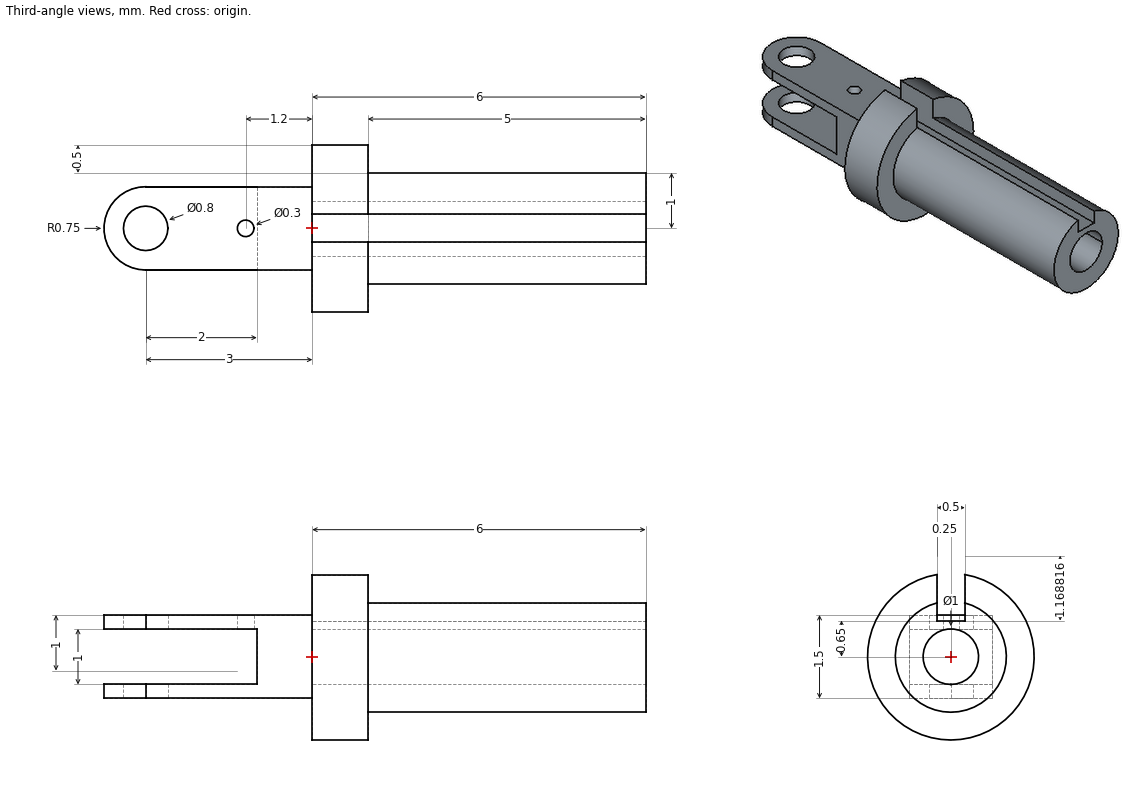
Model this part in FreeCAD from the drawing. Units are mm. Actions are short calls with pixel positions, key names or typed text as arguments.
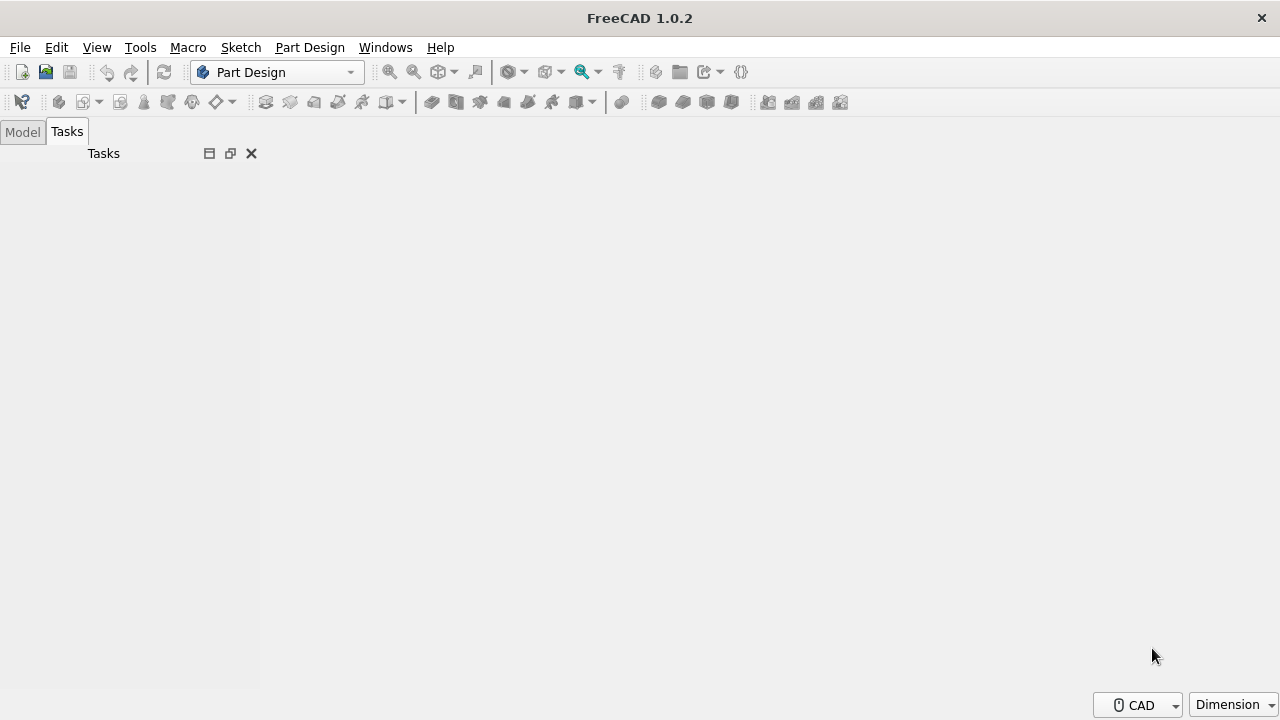
click(22, 72)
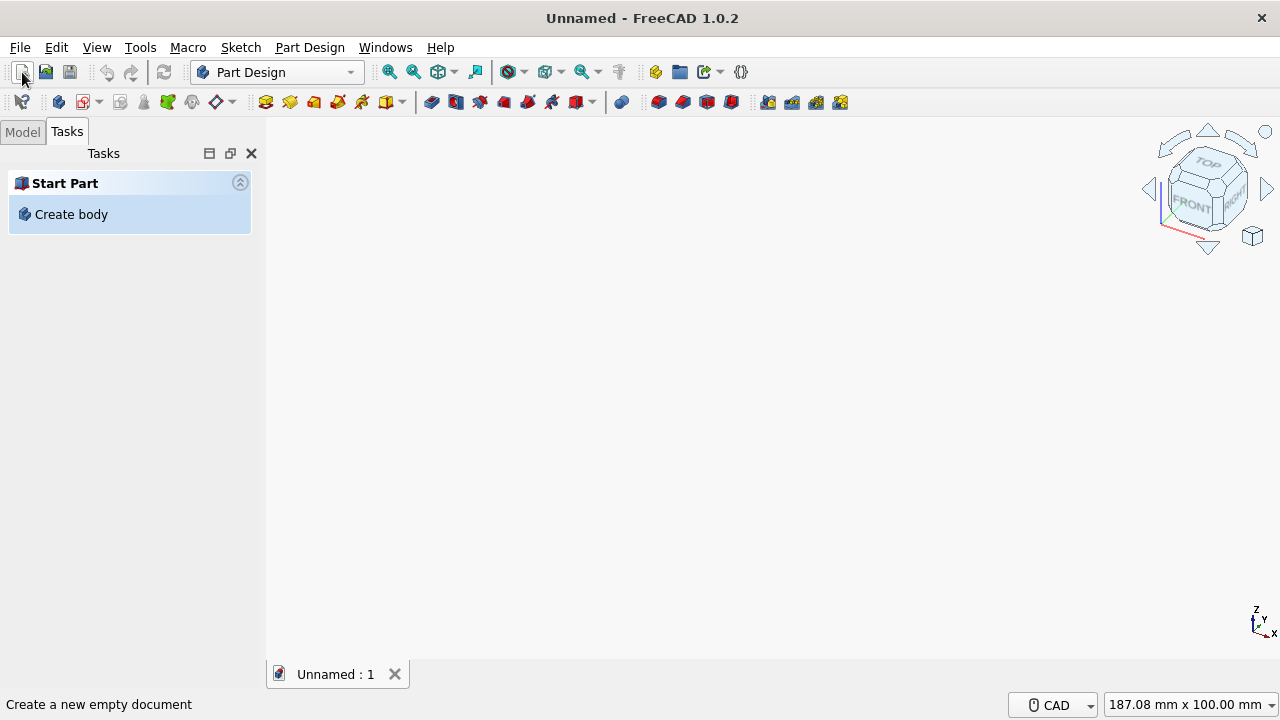
click(84, 102)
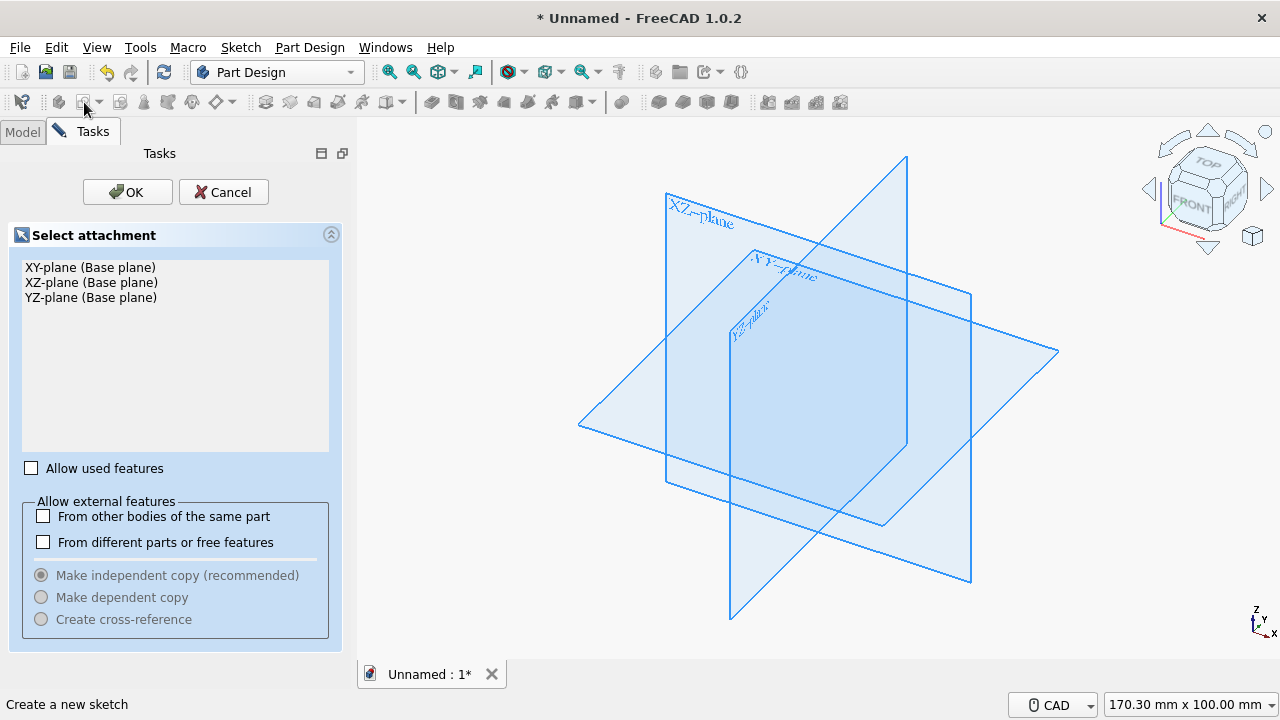
click(82, 268)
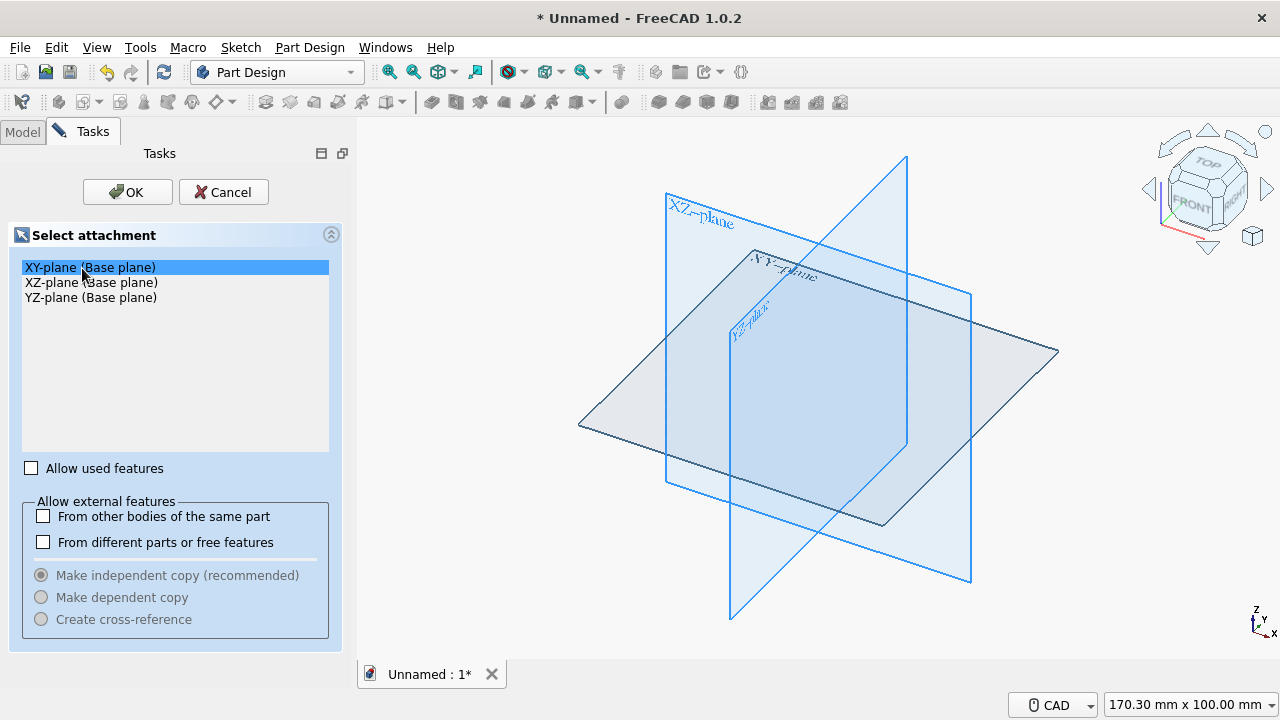
click(128, 192)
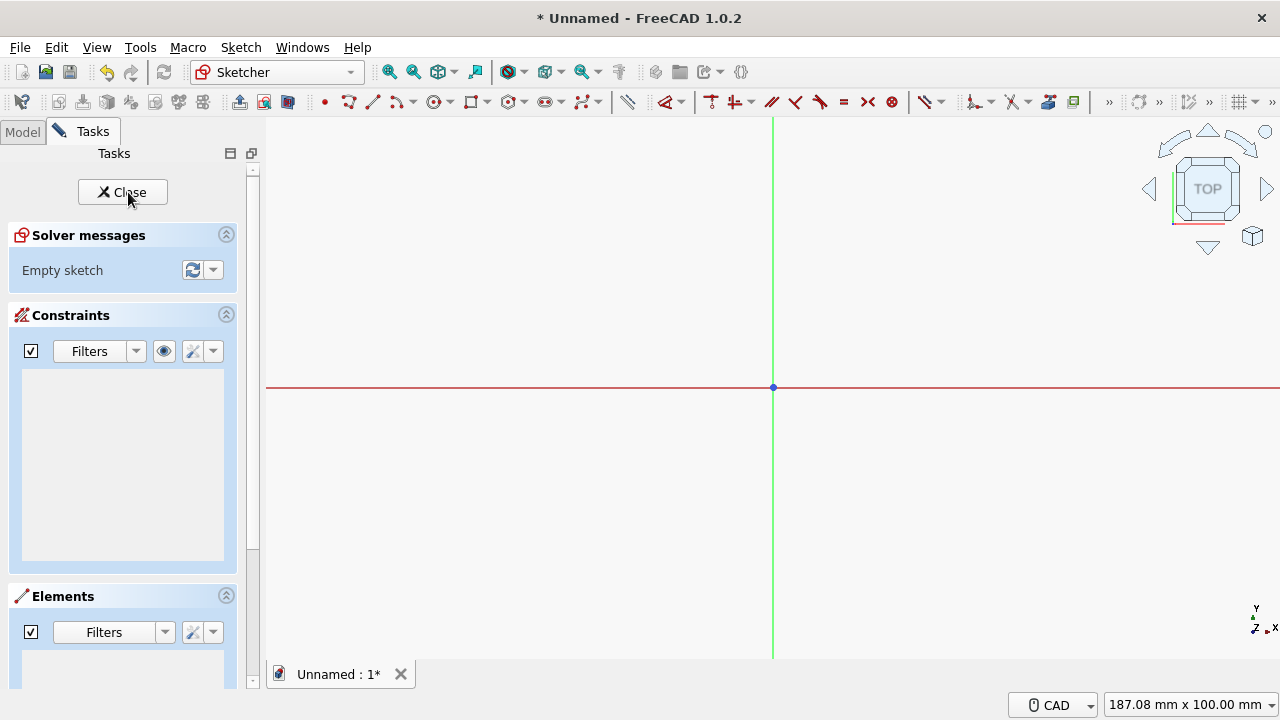
scroll(795, 384, up, 14)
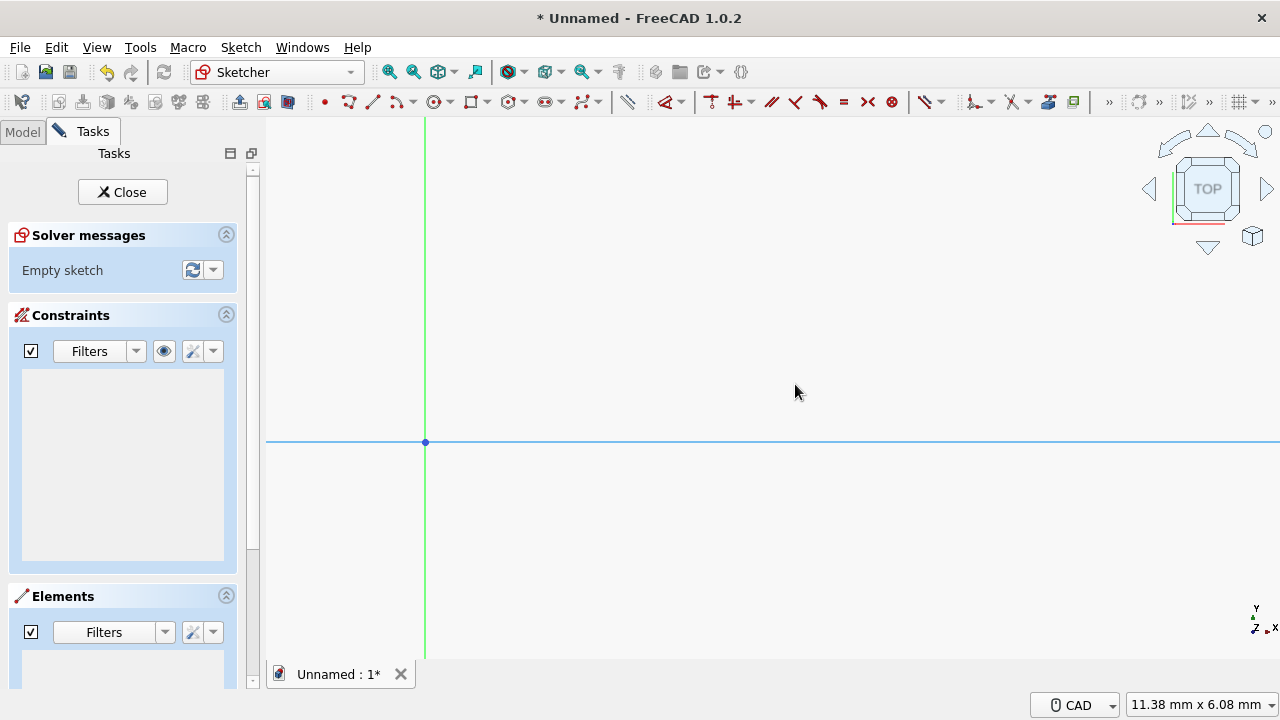
click(350, 102)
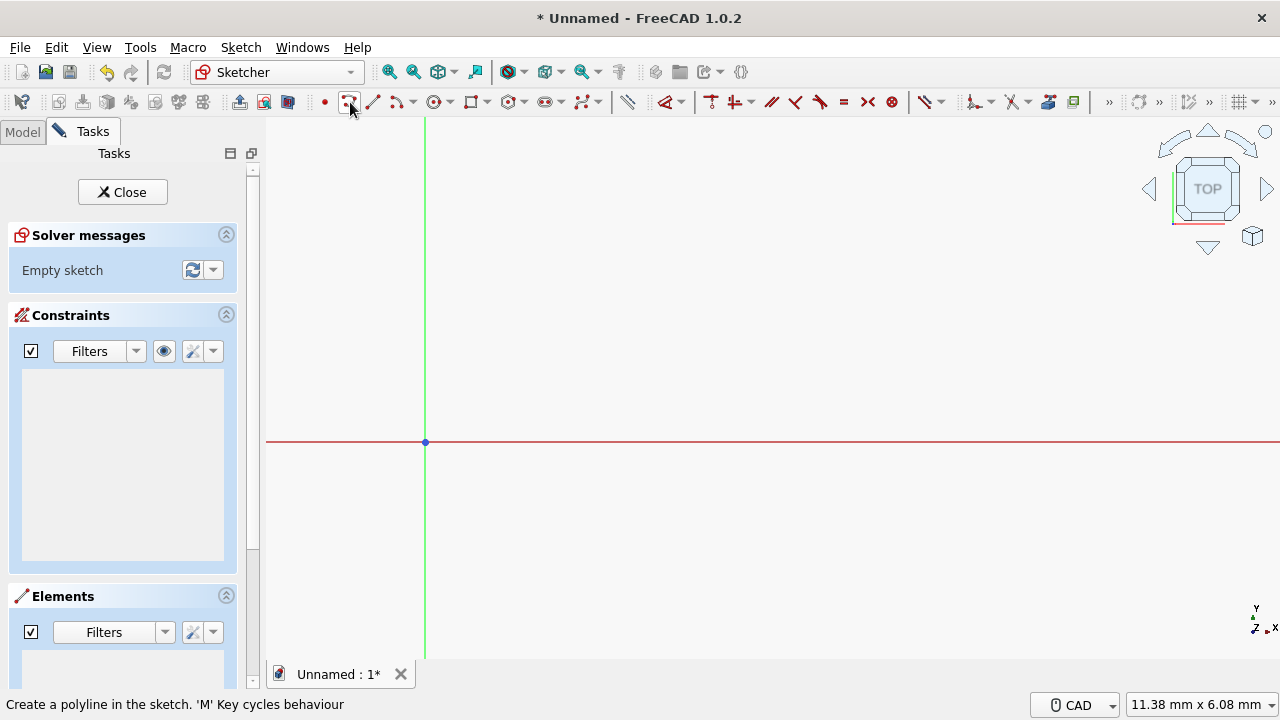
click(425, 442)
click(960, 433)
click(960, 353)
click(514, 353)
click(514, 308)
click(434, 308)
click(425, 442)
key(Escape)
key(Escape)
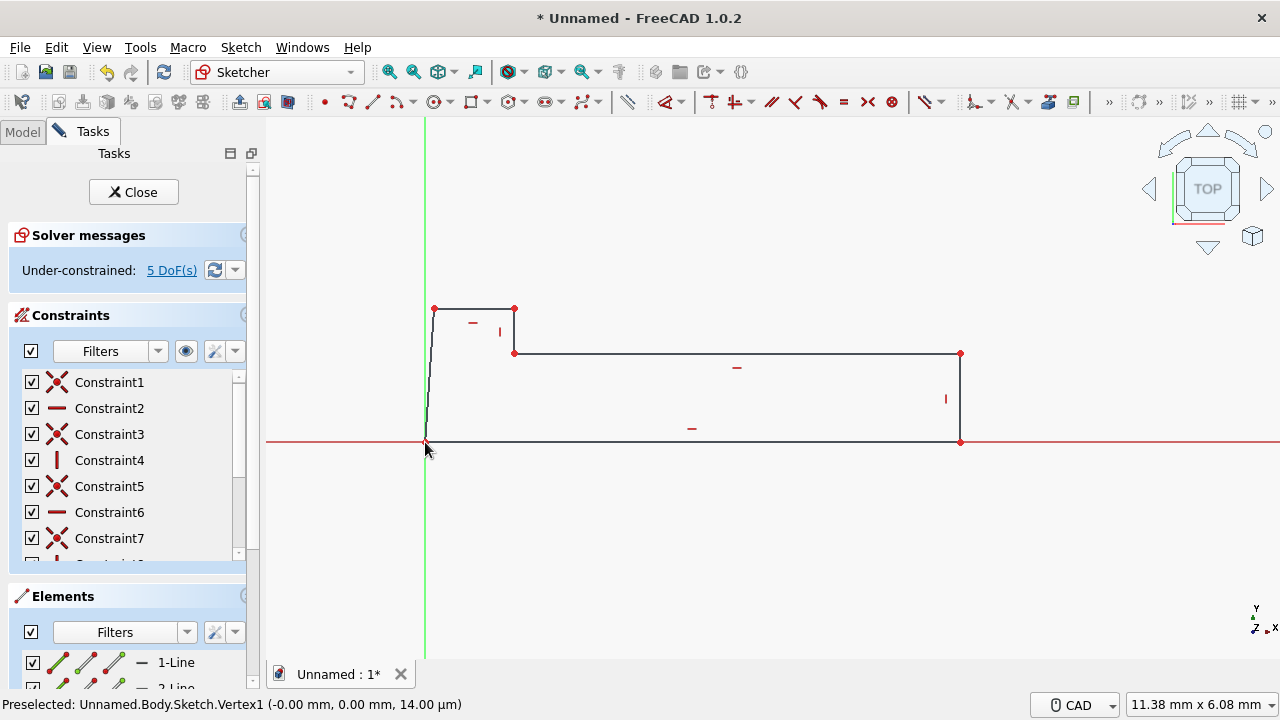
click(428, 402)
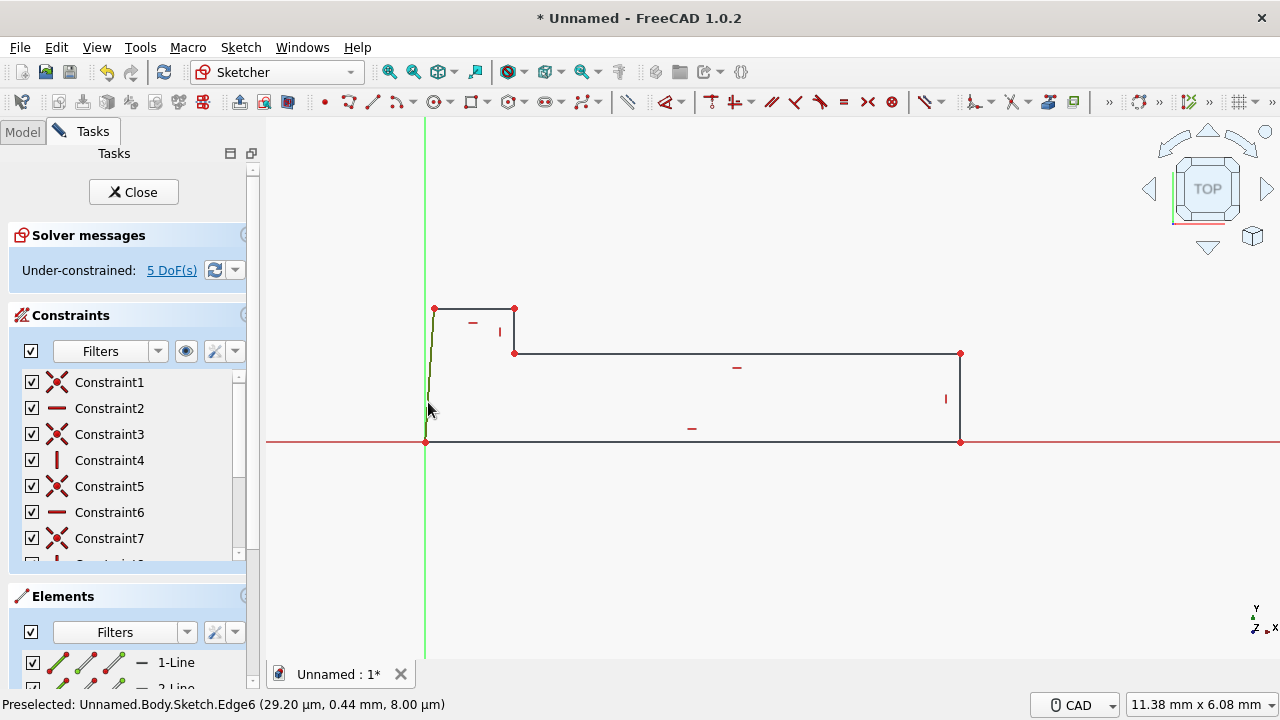
click(754, 102)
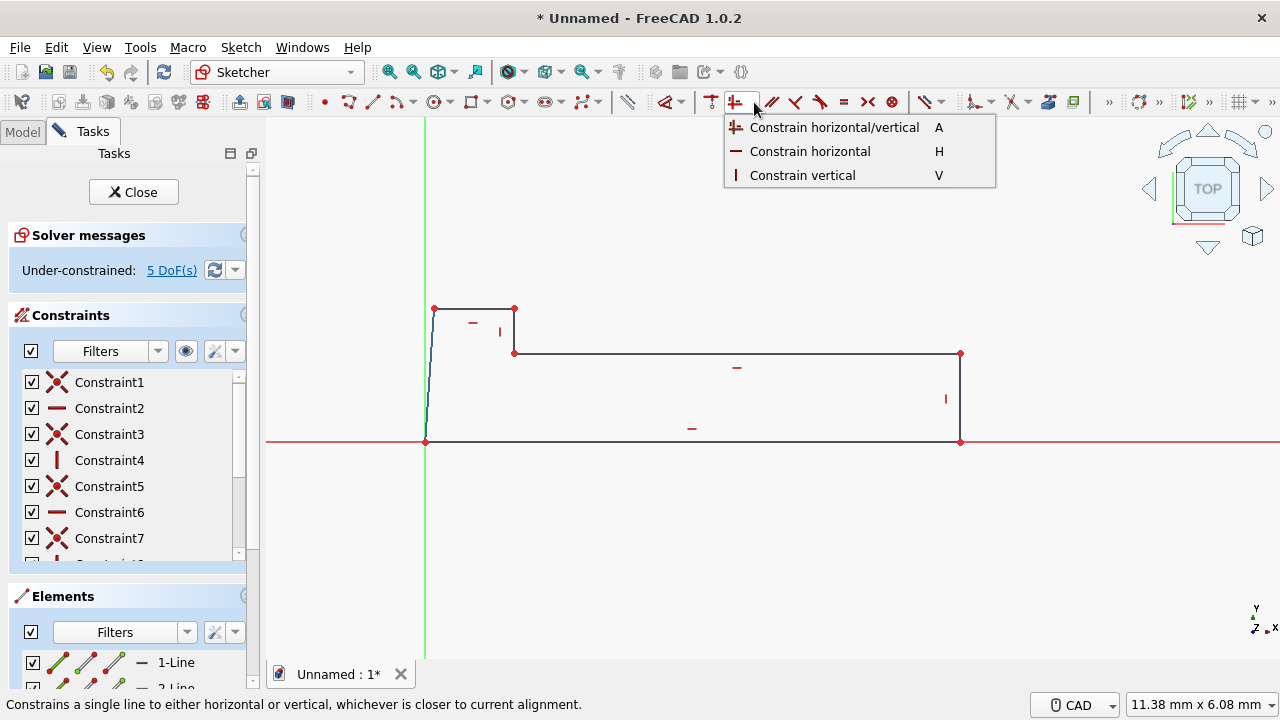
click(860, 175)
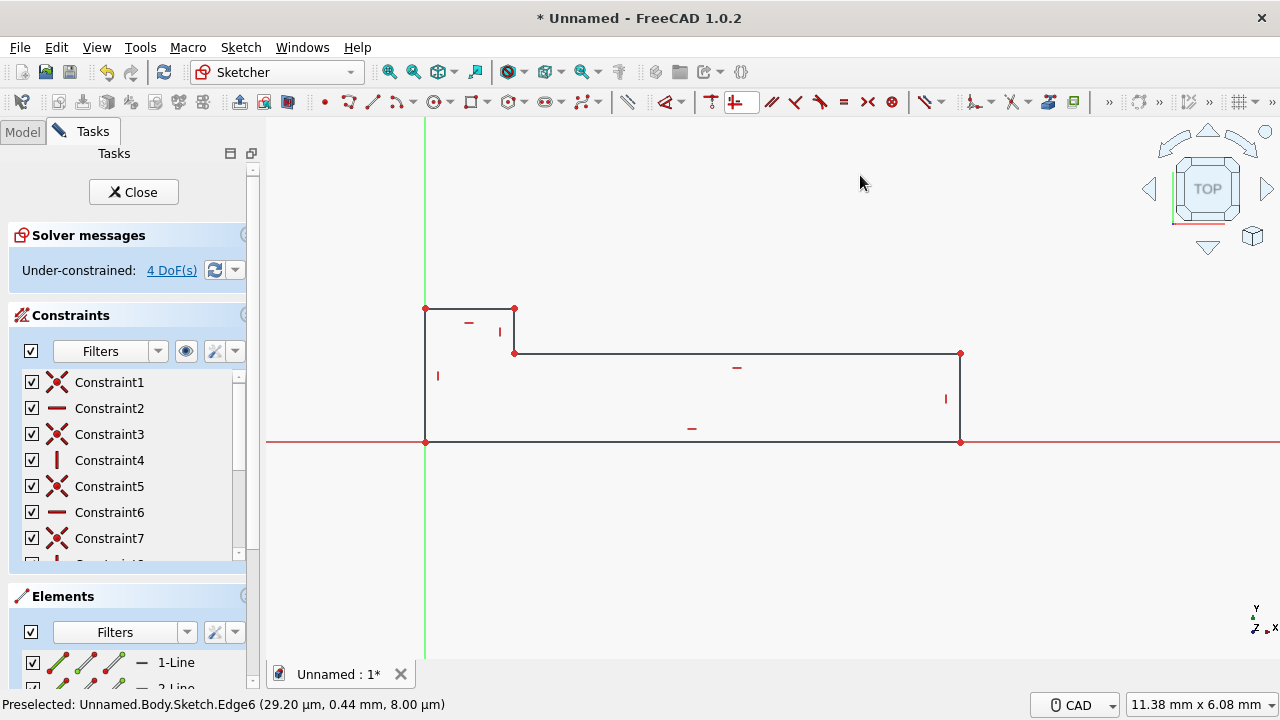
click(666, 102)